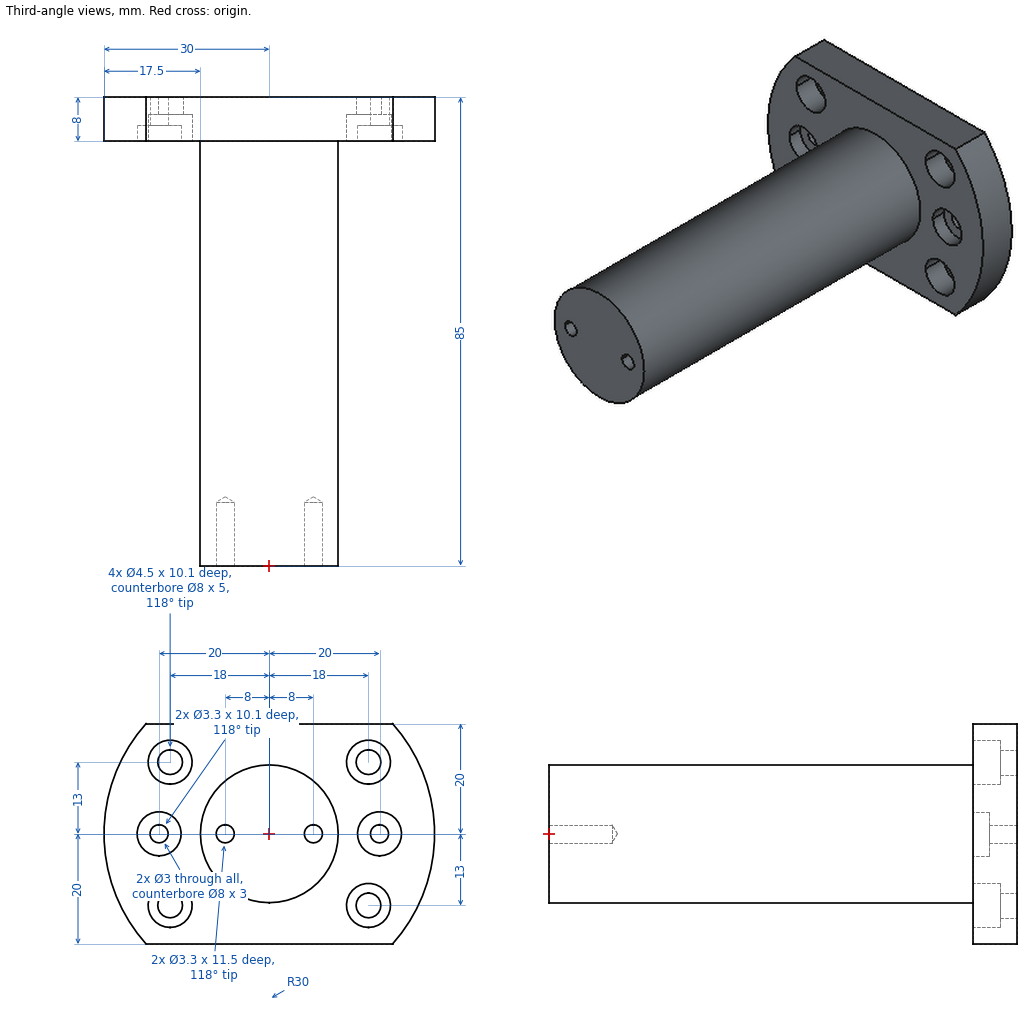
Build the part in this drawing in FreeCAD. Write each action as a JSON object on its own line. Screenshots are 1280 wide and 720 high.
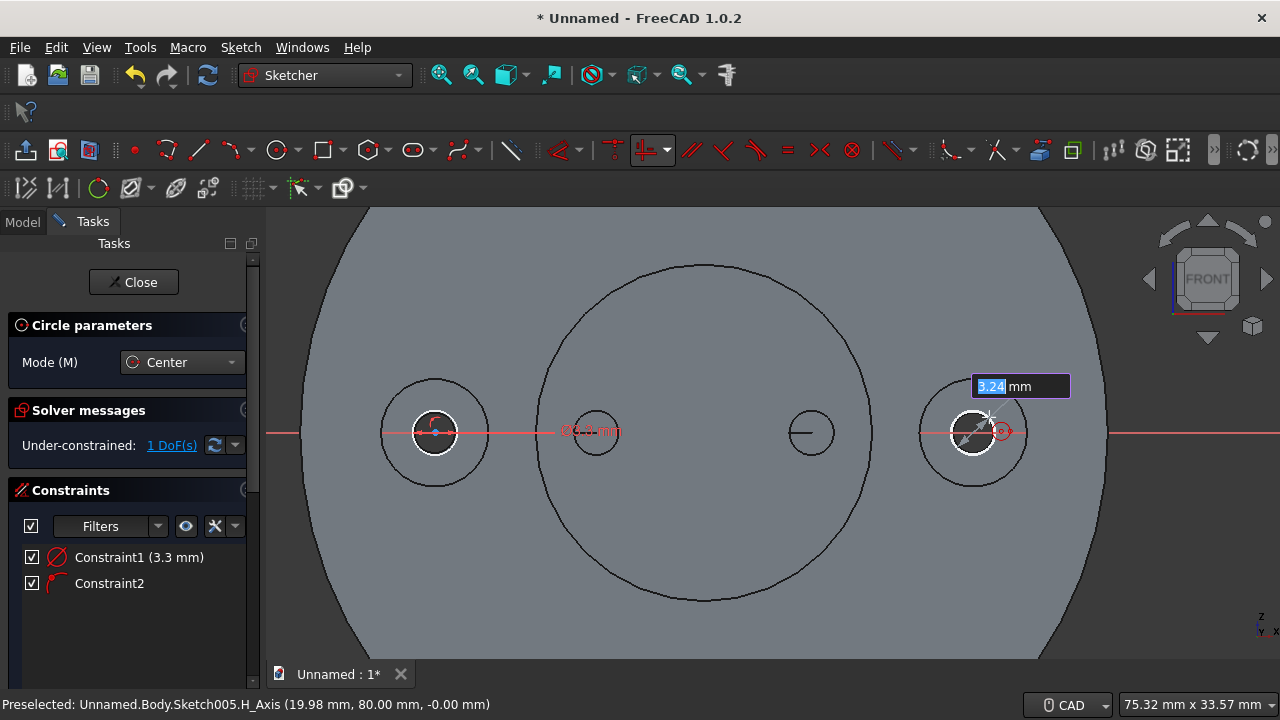
{"action": "type", "text": "3.3"}
{"action": "key", "text": "Return"}
{"action": "key", "text": "Escape"}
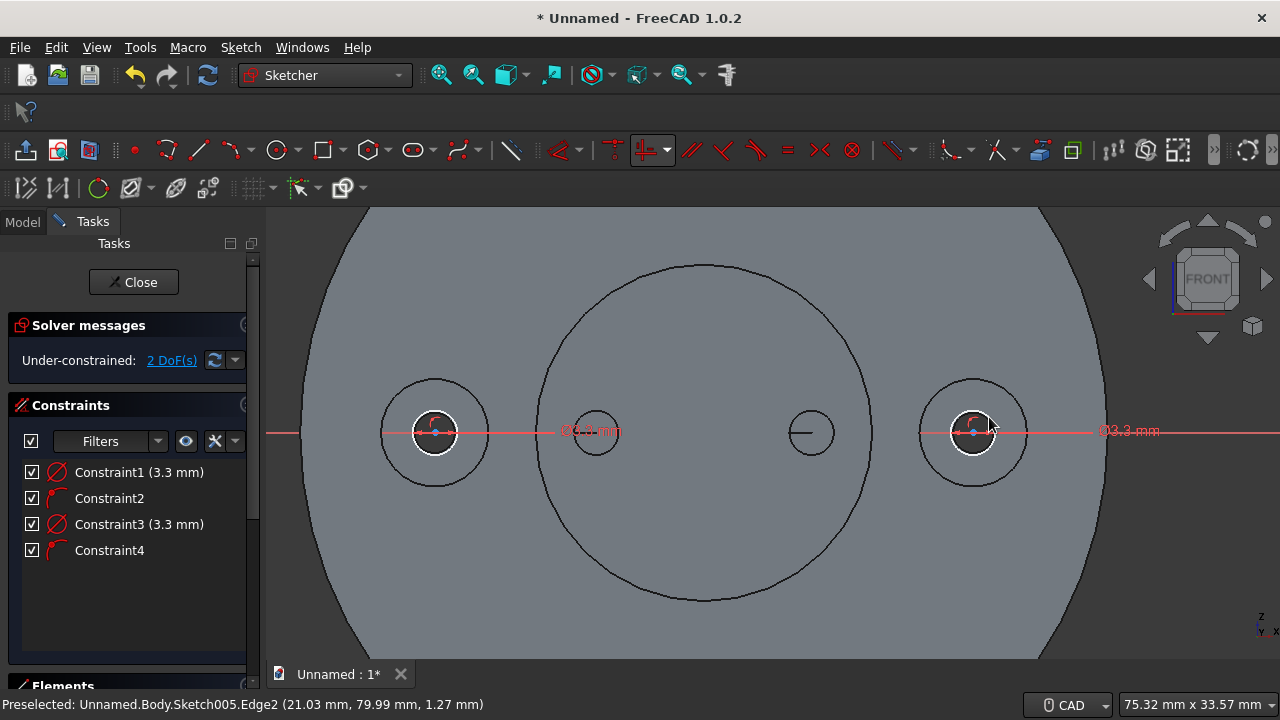
{"action": "left_click", "coordinate": [558, 150]}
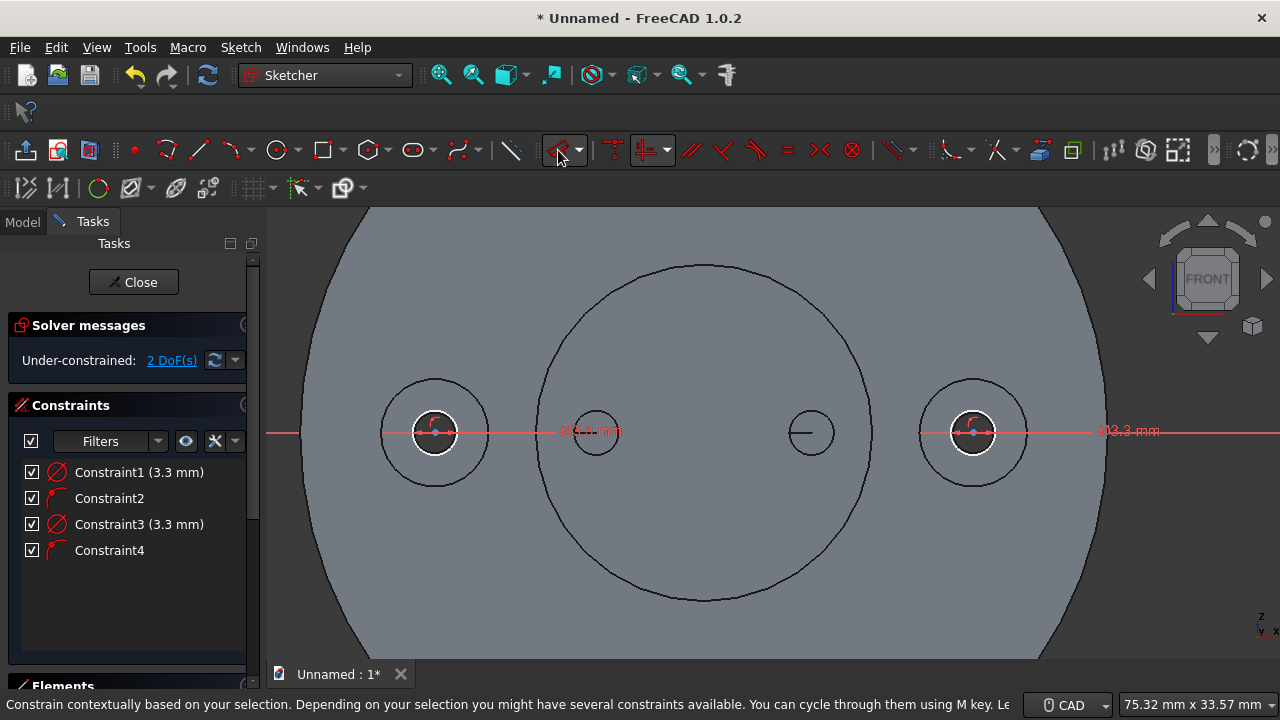
{"action": "left_click", "coordinate": [435, 433]}
{"action": "left_click", "coordinate": [570, 467]}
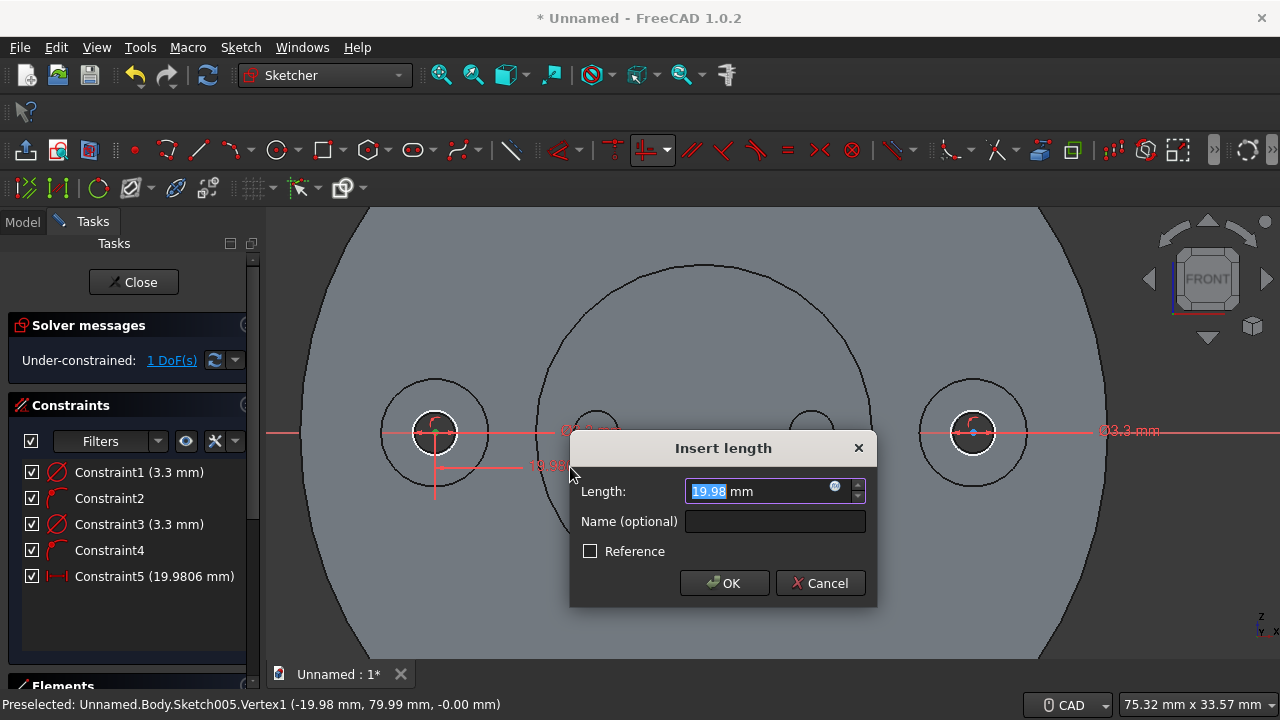
{"action": "type", "text": "20"}
{"action": "key", "text": "Return"}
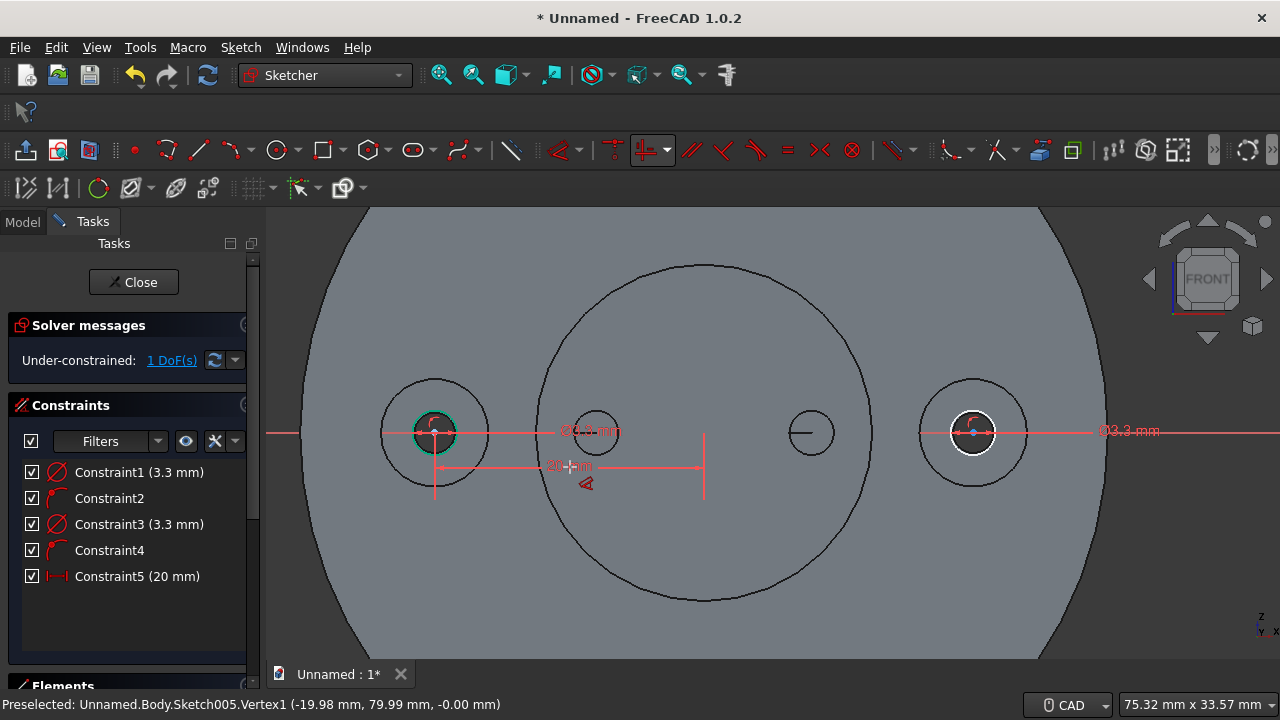
{"action": "left_click", "coordinate": [973, 433]}
{"action": "left_click", "coordinate": [839, 467]}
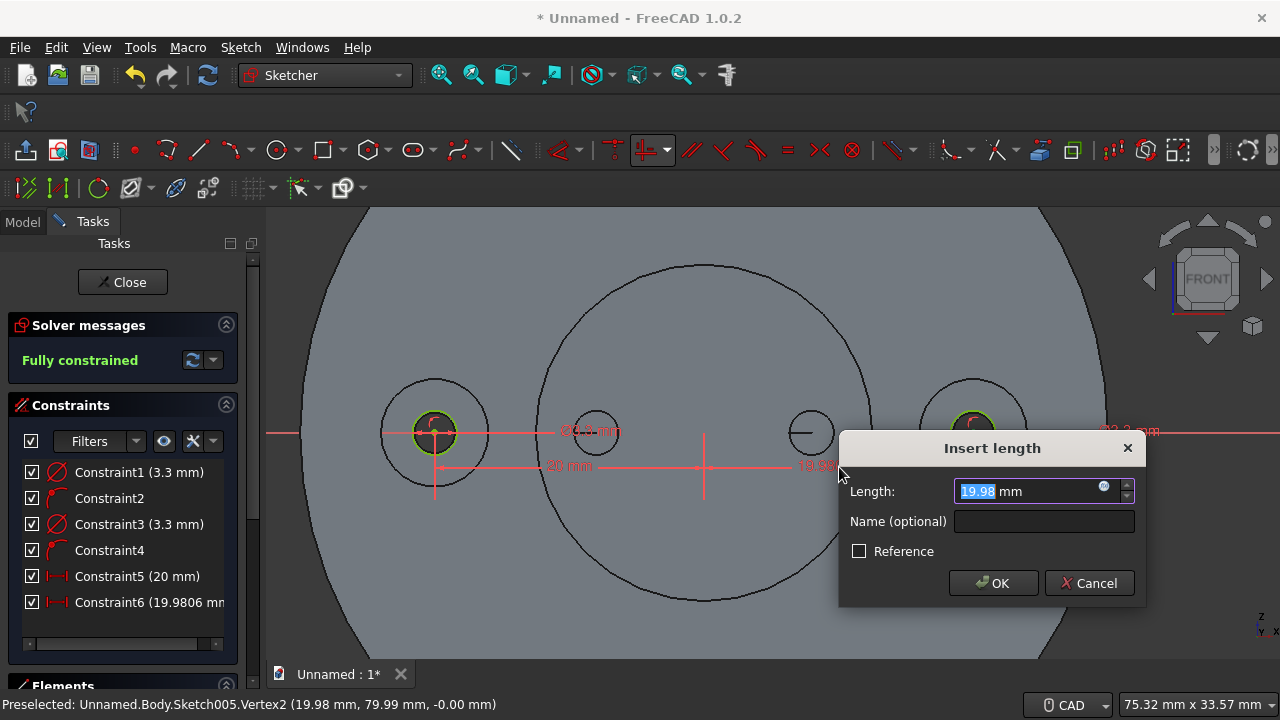
{"action": "type", "text": "20"}
{"action": "key", "text": "Return"}
{"action": "key", "text": "Escape"}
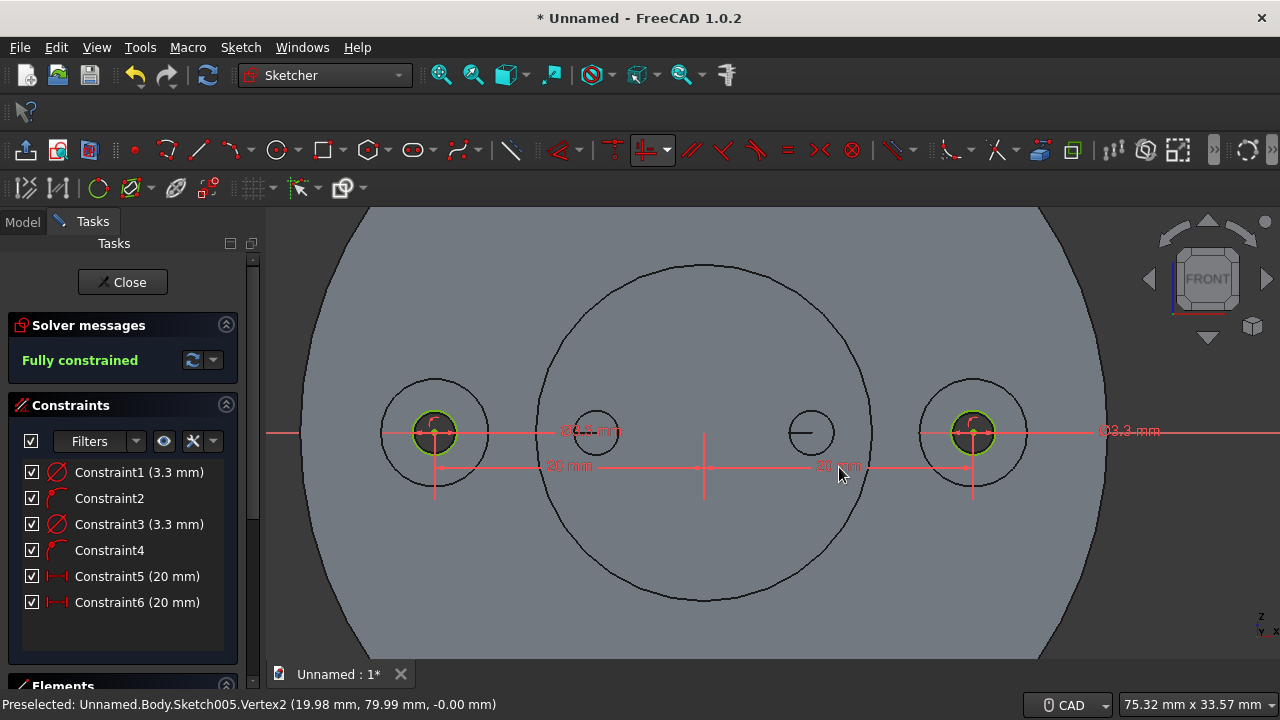
{"action": "left_click", "coordinate": [123, 282]}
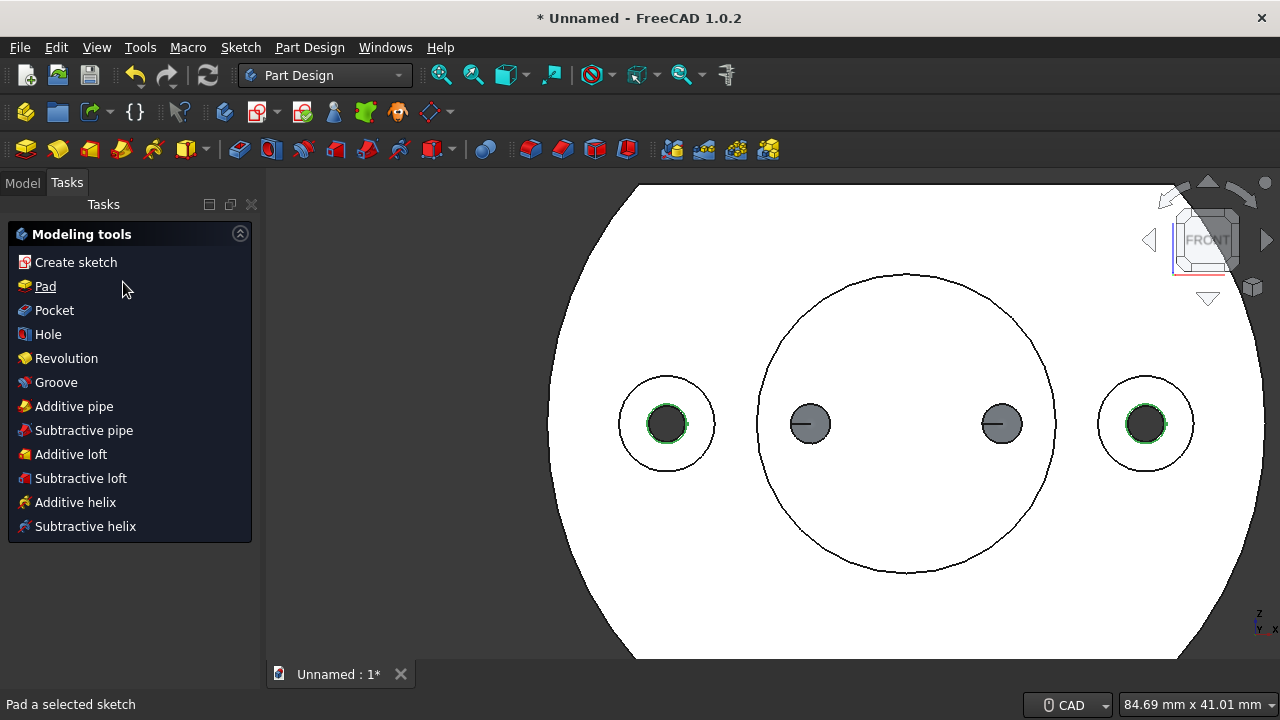
{"action": "left_click", "coordinate": [272, 150]}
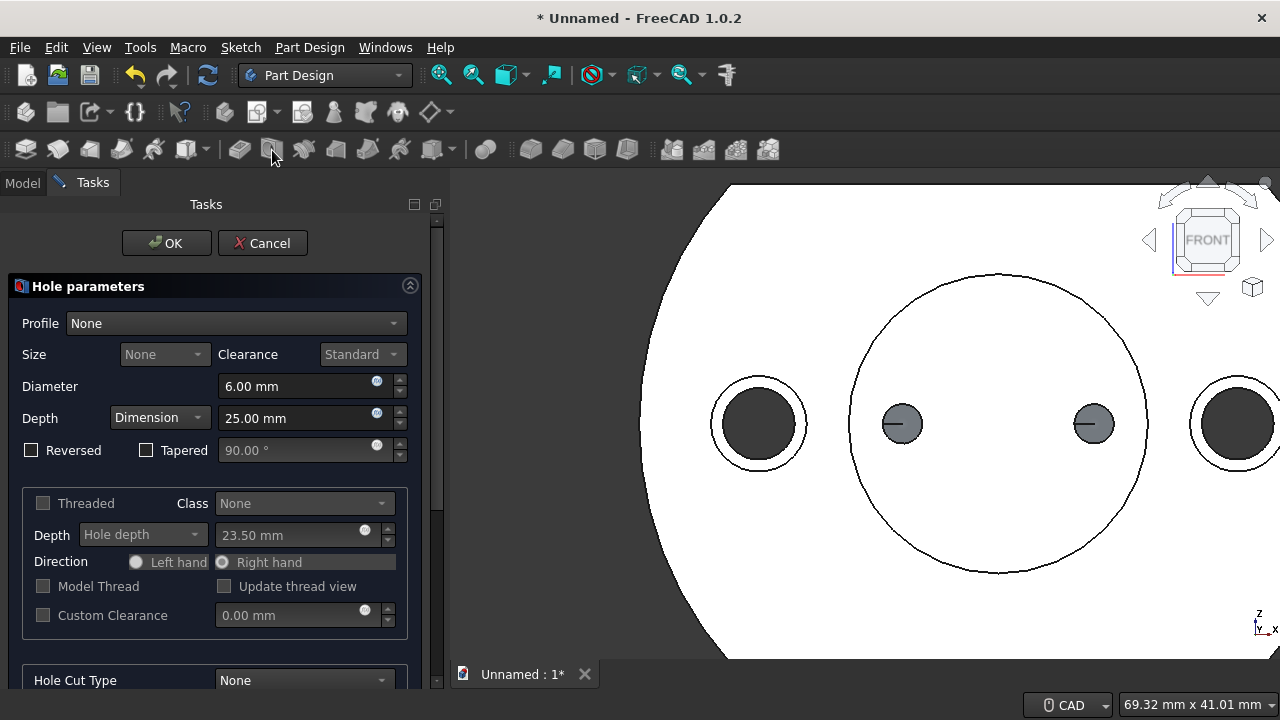
{"action": "triple_click", "coordinate": [305, 386]}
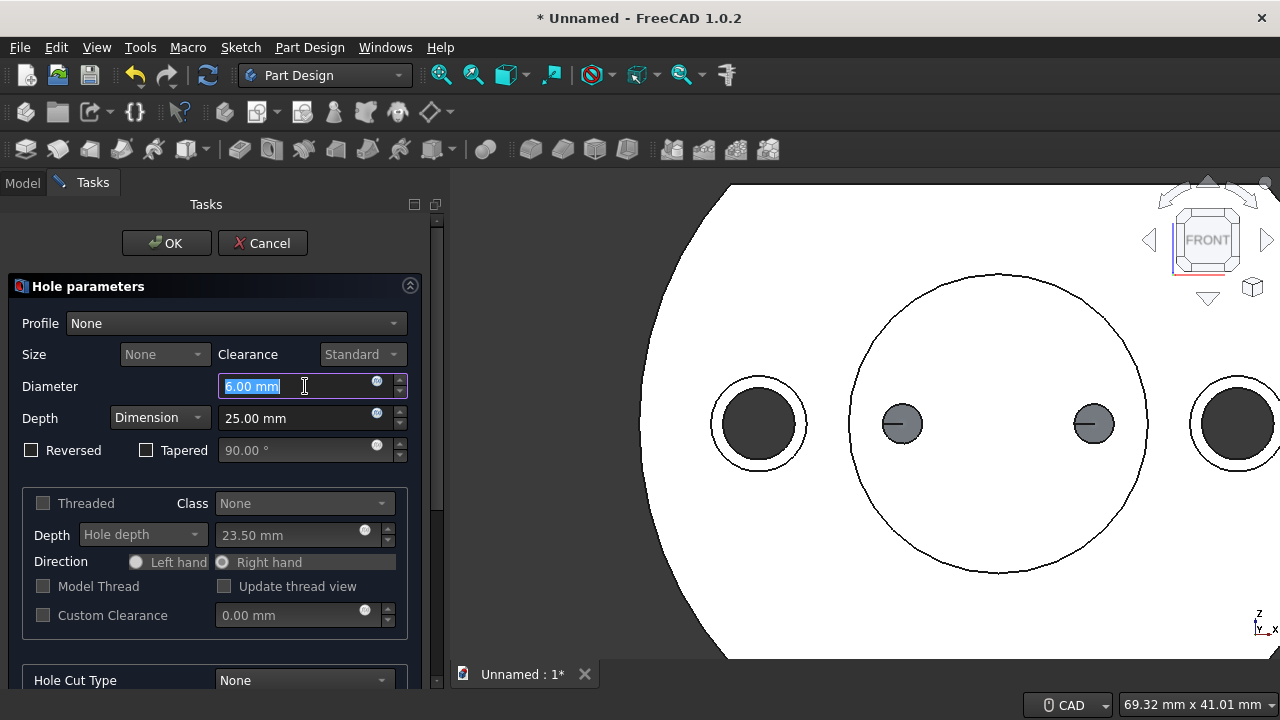
{"action": "type", "text": "3.3"}
{"action": "key", "text": "Tab"}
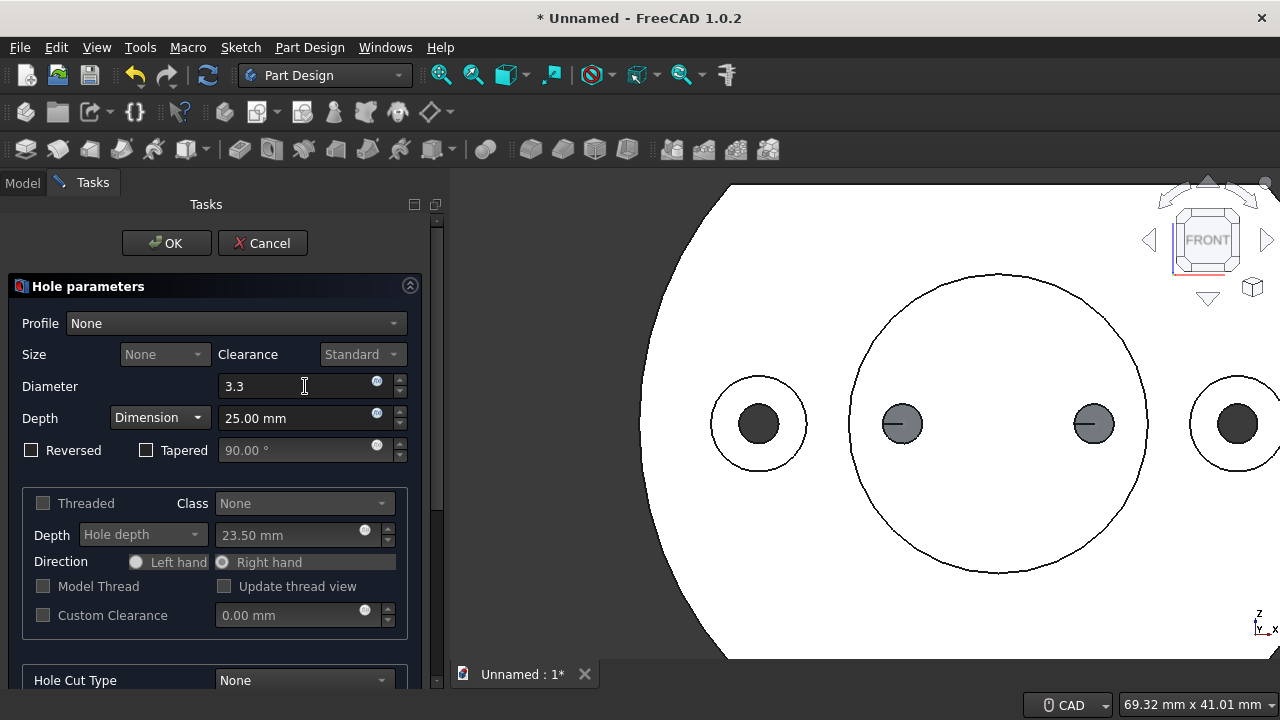
{"action": "triple_click", "coordinate": [305, 418]}